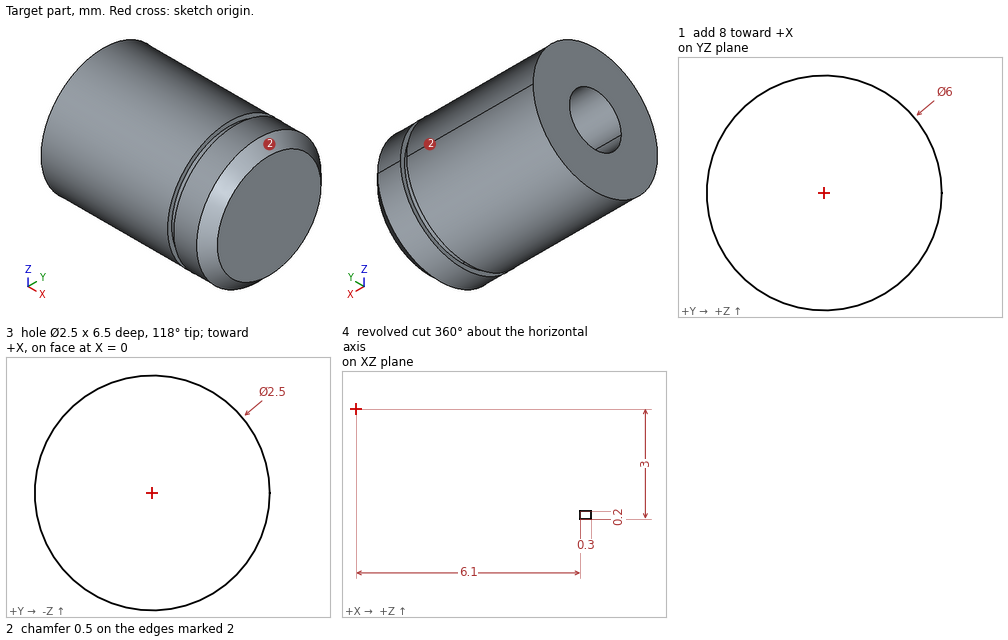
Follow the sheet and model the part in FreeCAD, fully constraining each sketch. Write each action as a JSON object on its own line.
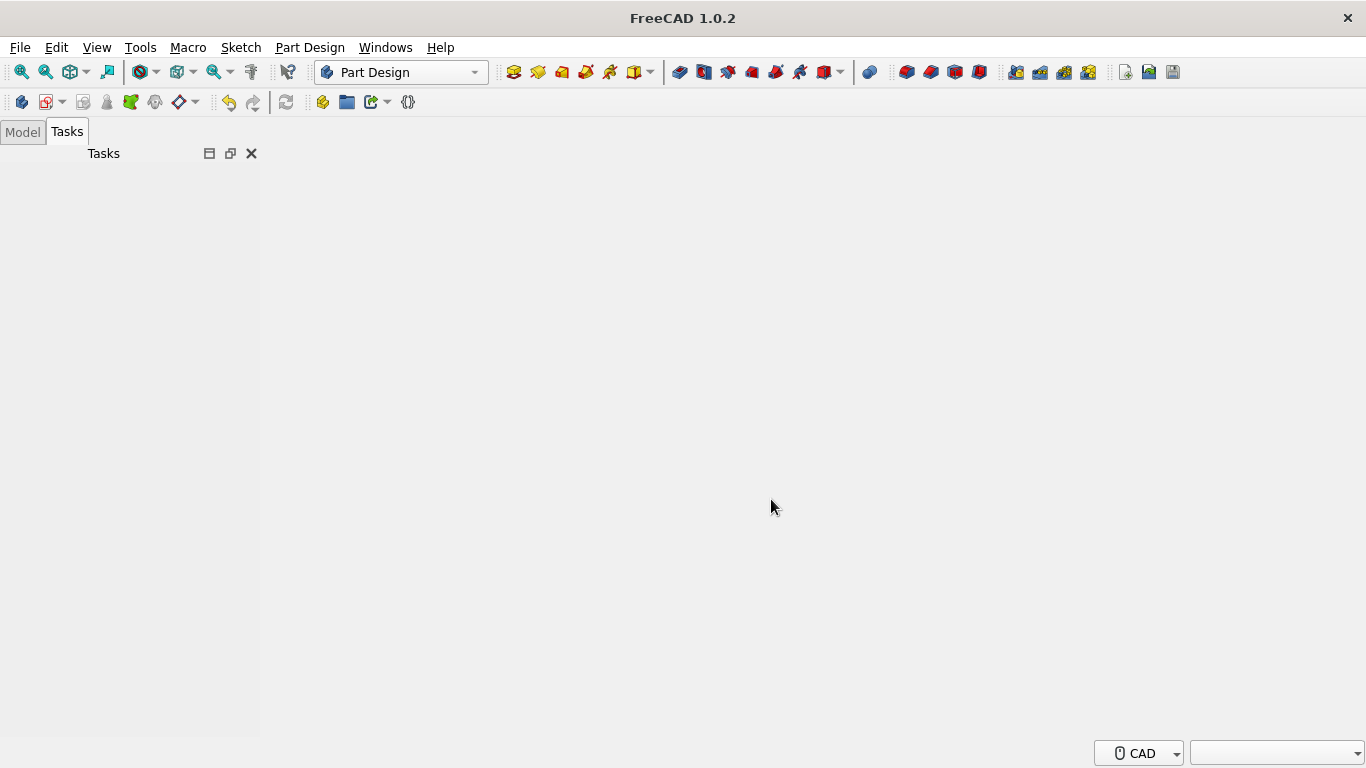
{"action": "left_click", "coordinate": [1126, 72]}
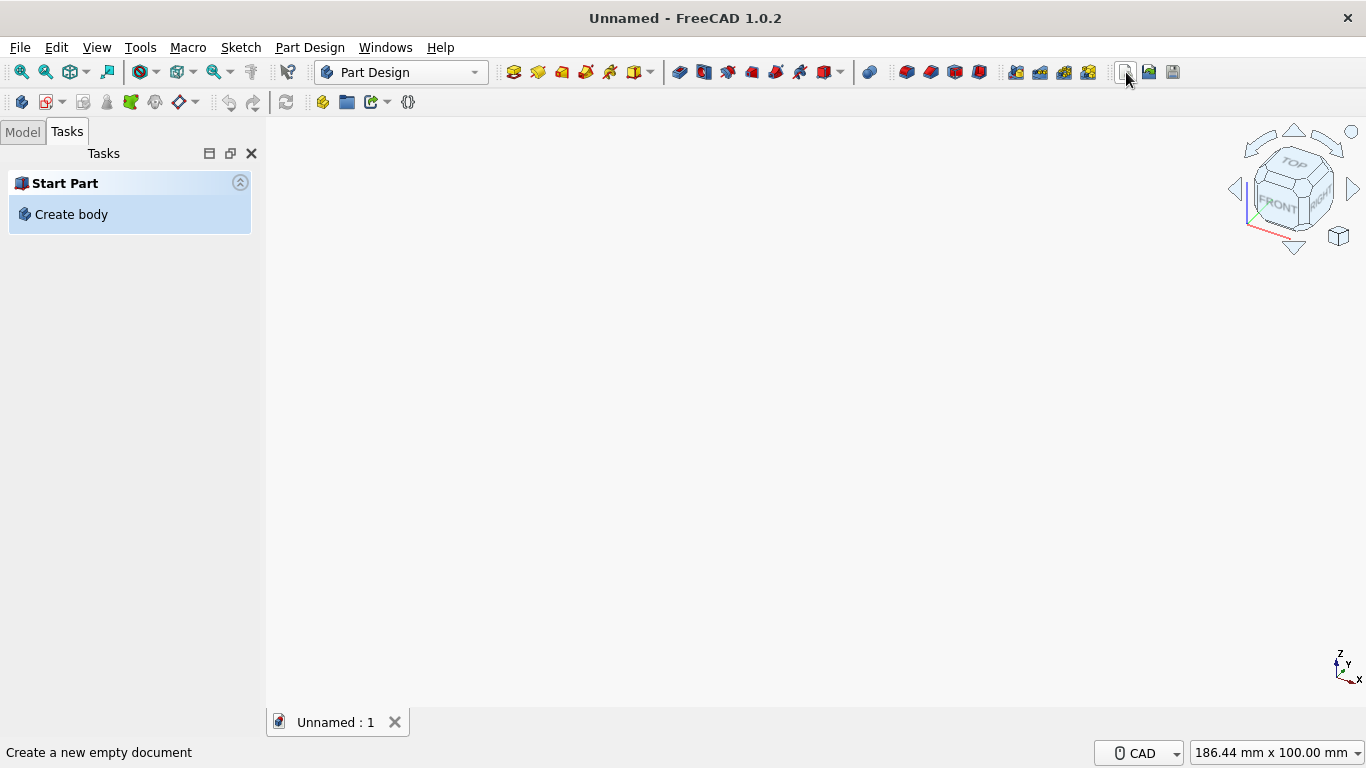
{"action": "left_click", "coordinate": [46, 102]}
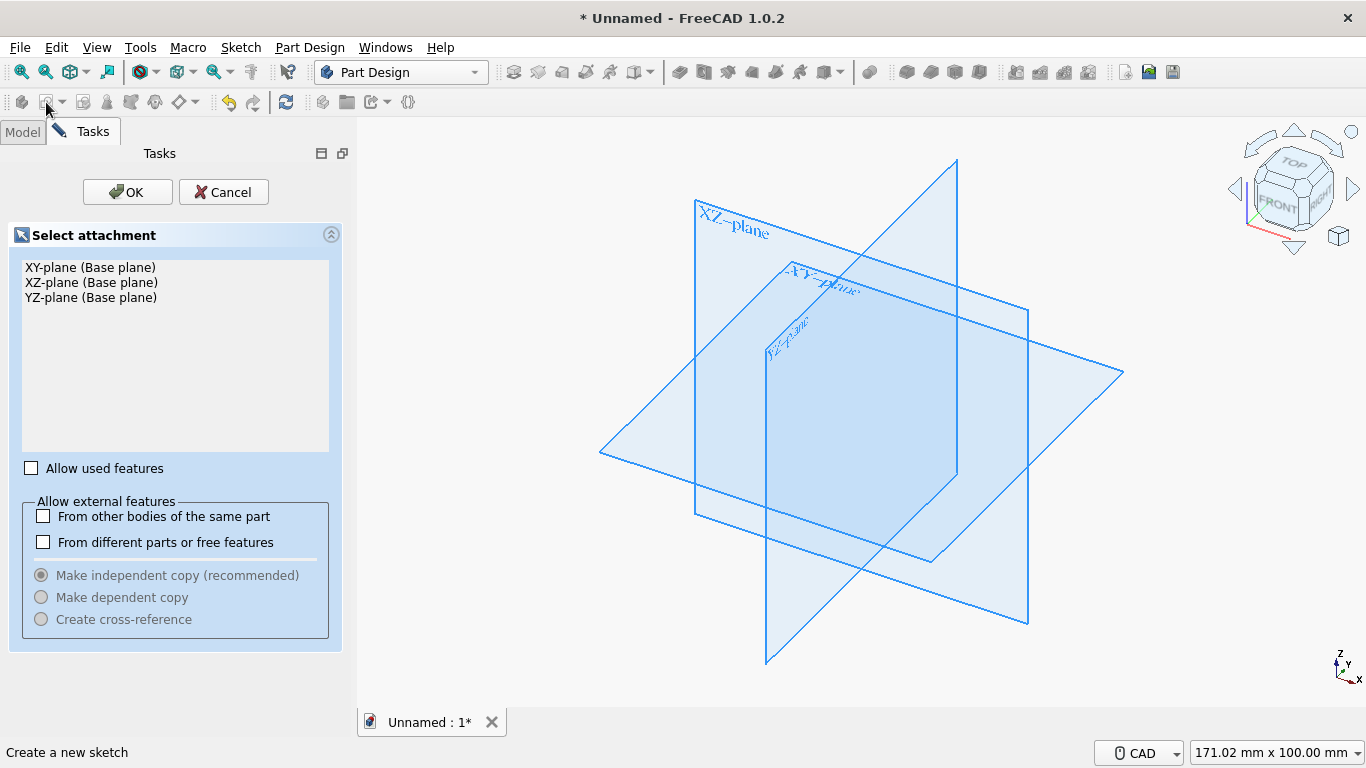
{"action": "left_click", "coordinate": [82, 298]}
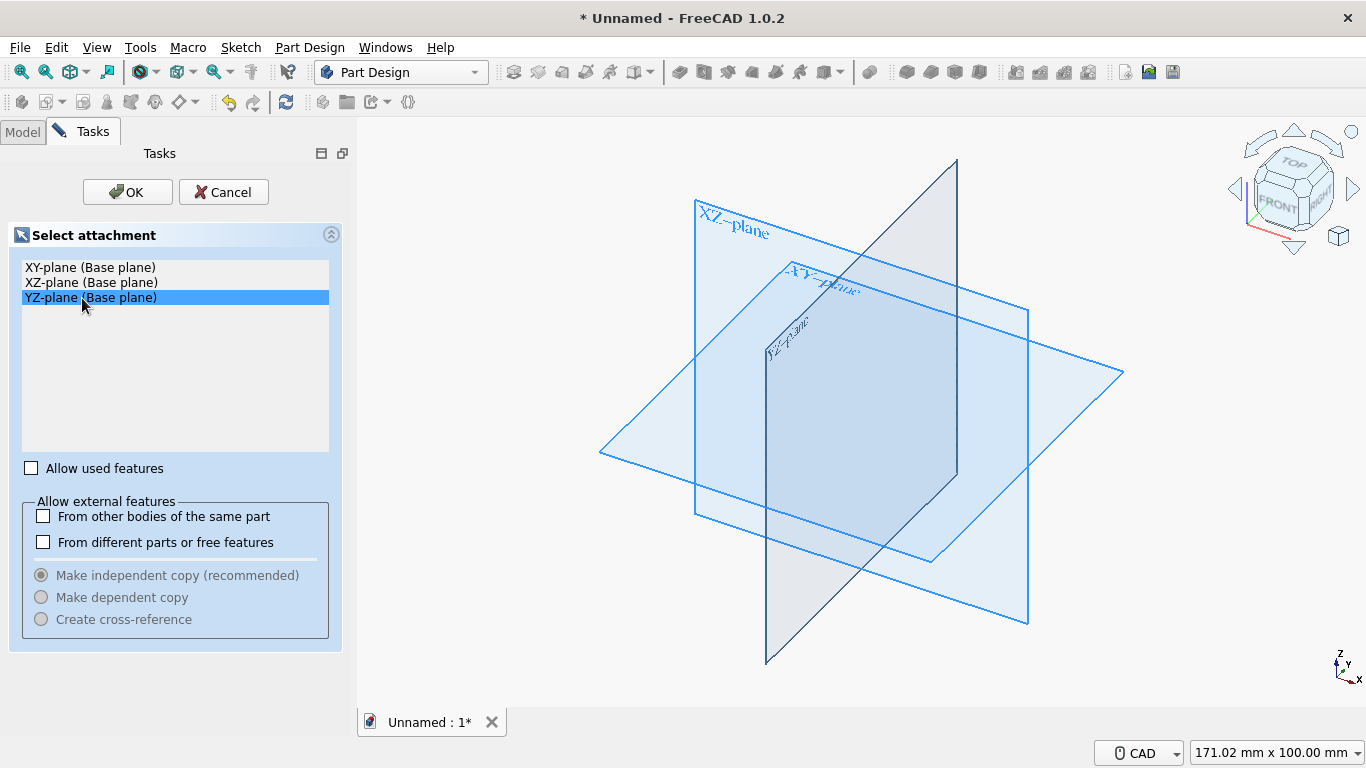
{"action": "left_click", "coordinate": [128, 192]}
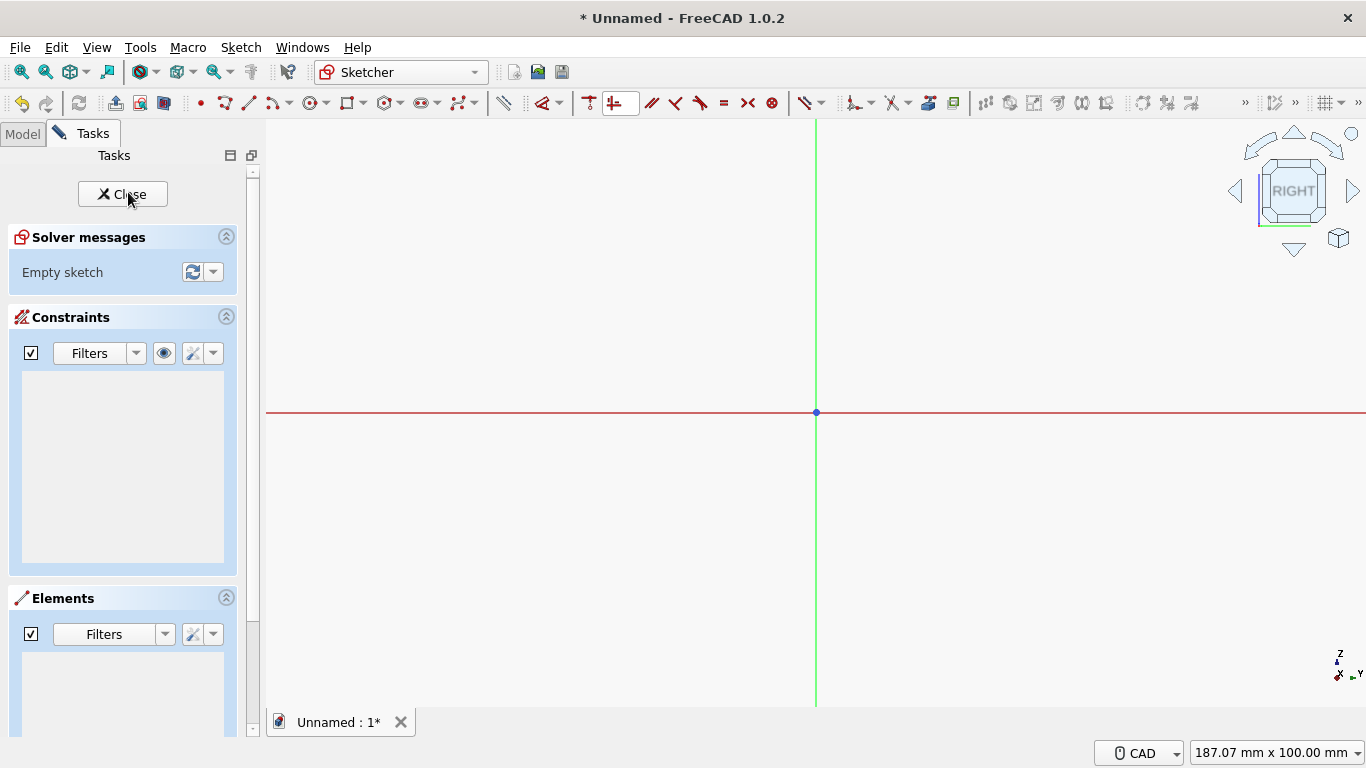
{"action": "scroll", "coordinate": [823, 413], "scroll_direction": "up", "scroll_amount": 12}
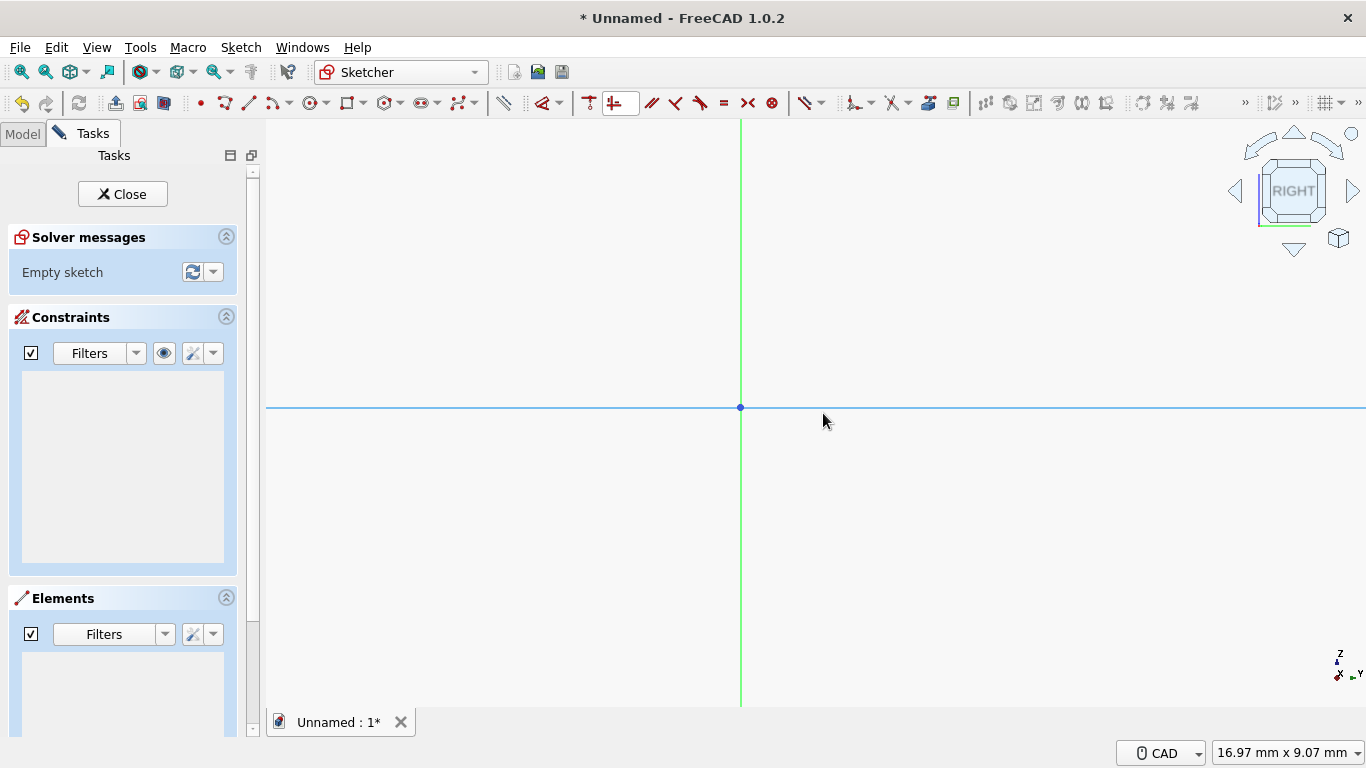
{"action": "left_click", "coordinate": [310, 104]}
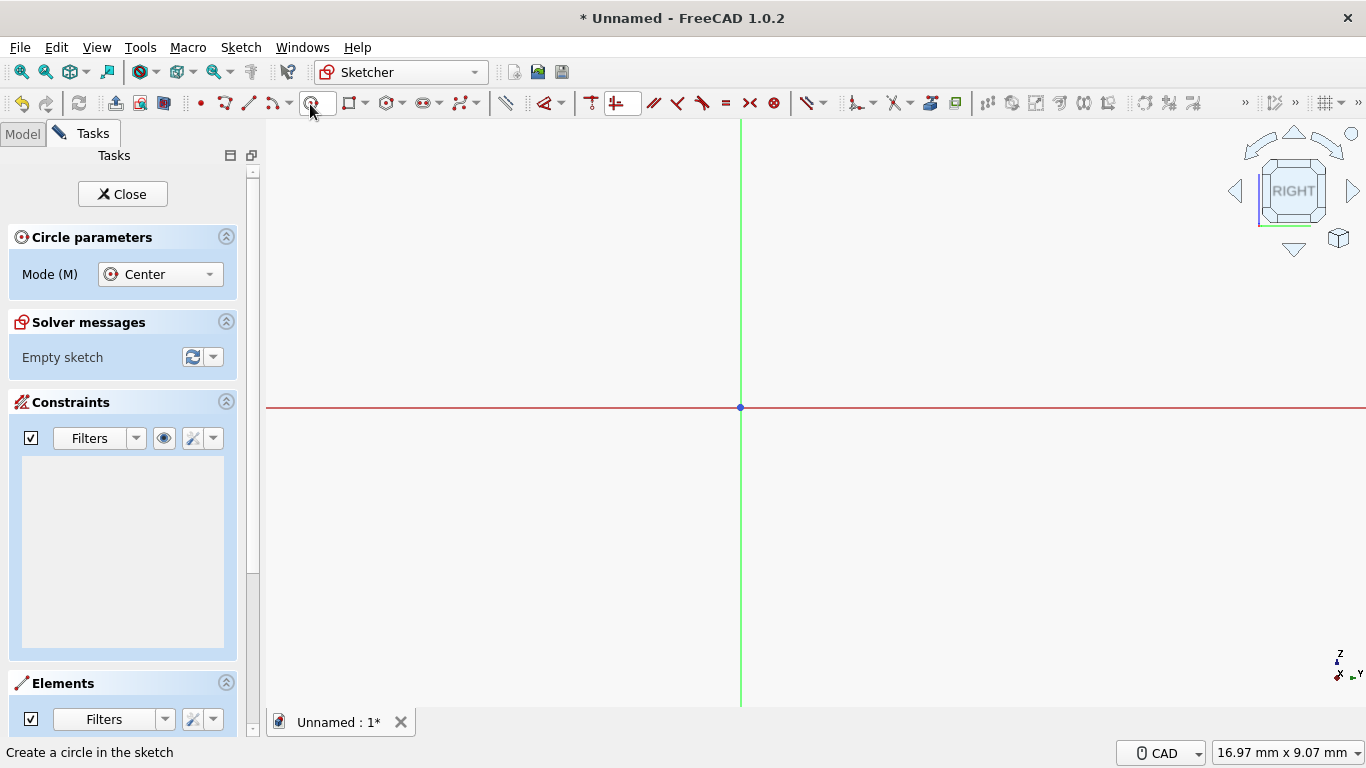
{"action": "left_click", "coordinate": [741, 408]}
{"action": "mouse_move", "coordinate": [878, 270]}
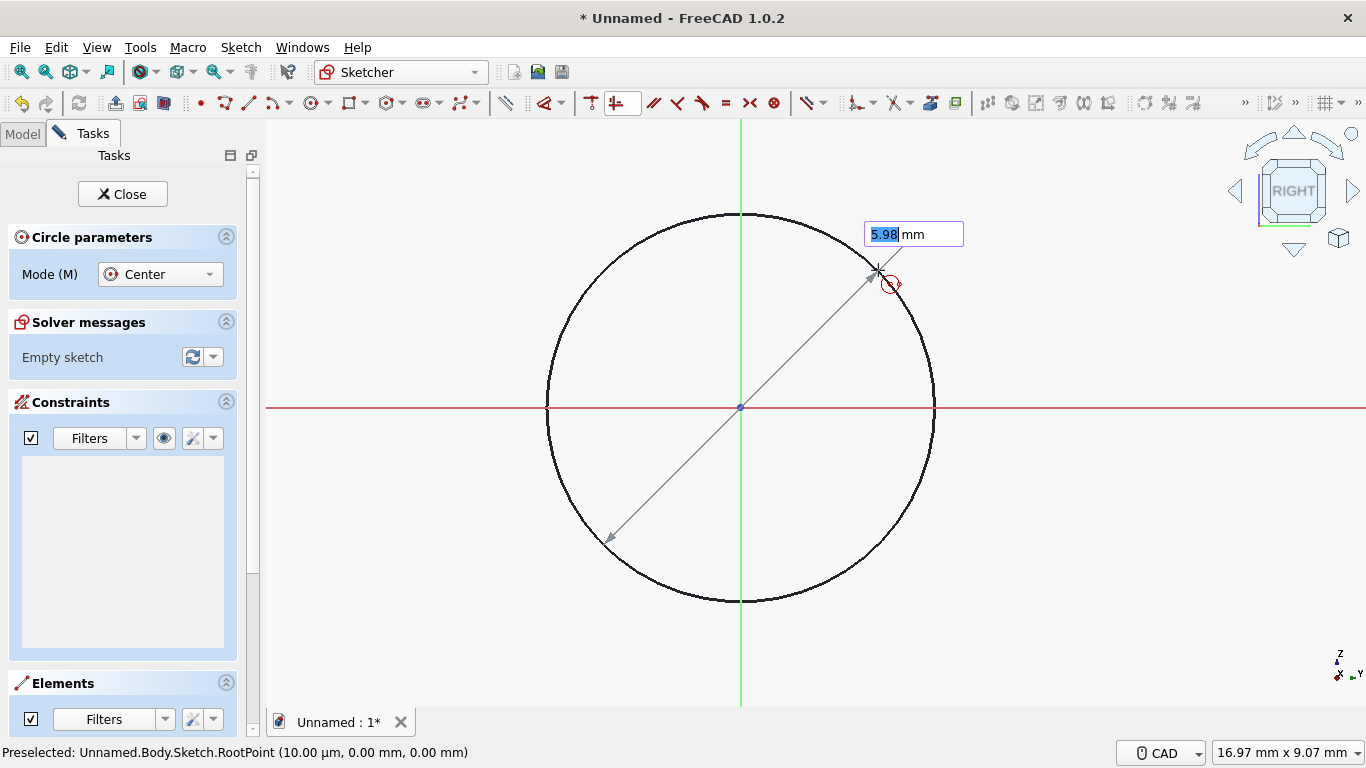
{"action": "type", "text": "6"}
{"action": "key", "text": "Return"}
{"action": "key", "text": "Escape"}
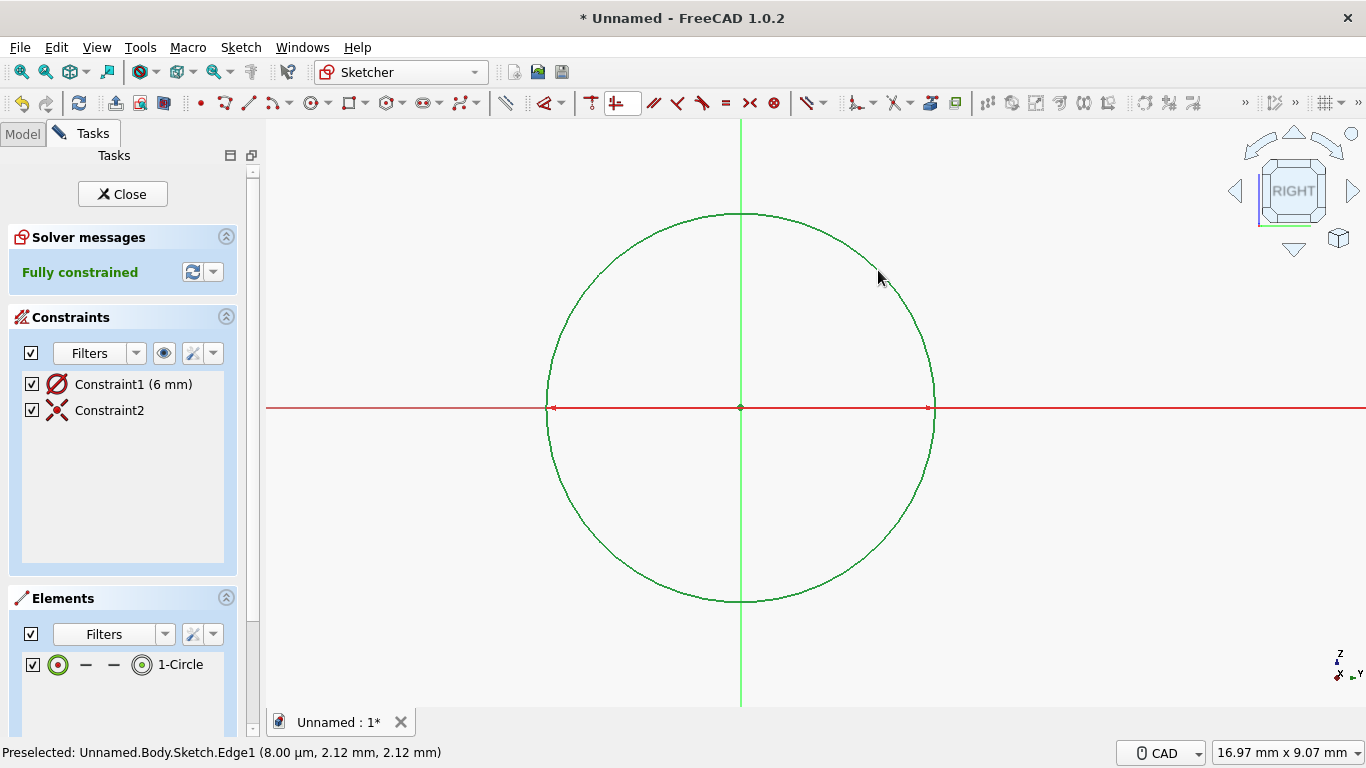
{"action": "left_click", "coordinate": [123, 194]}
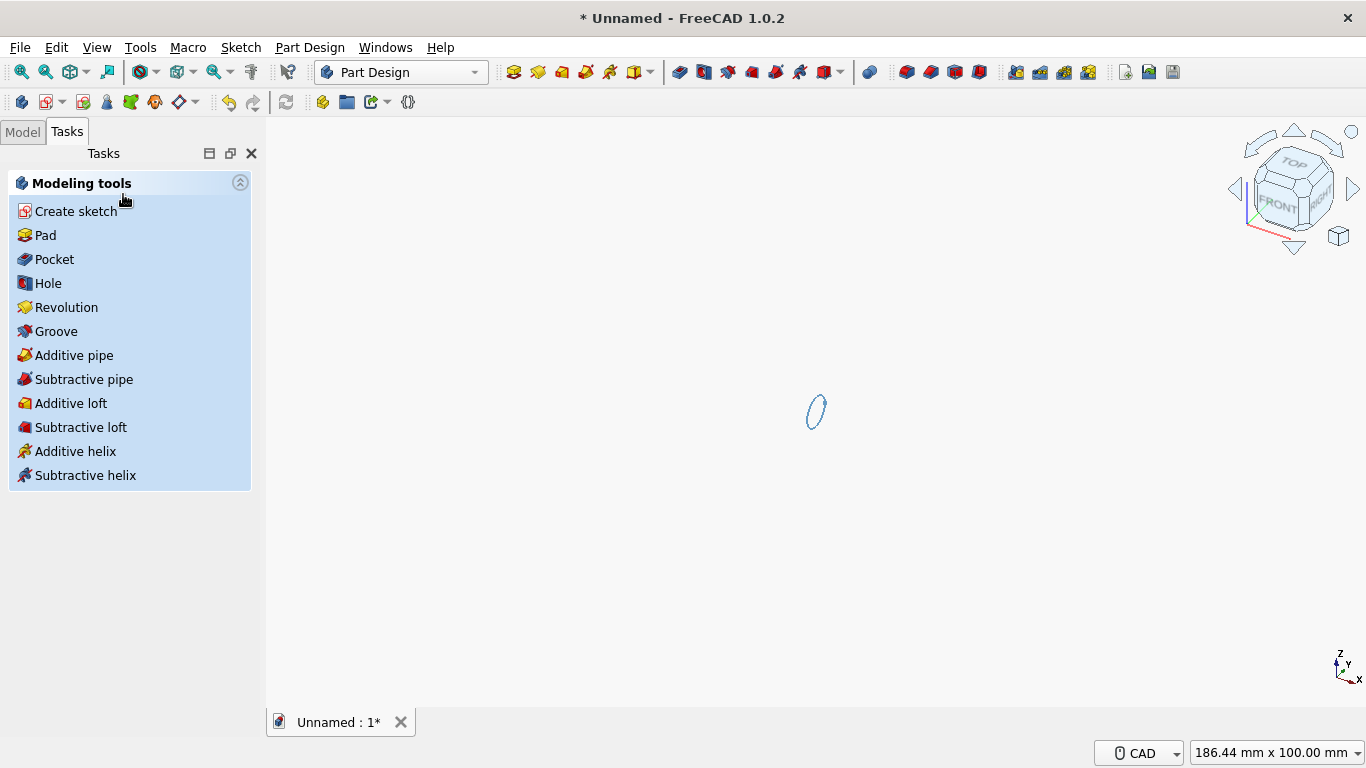
{"action": "left_click", "coordinate": [514, 72]}